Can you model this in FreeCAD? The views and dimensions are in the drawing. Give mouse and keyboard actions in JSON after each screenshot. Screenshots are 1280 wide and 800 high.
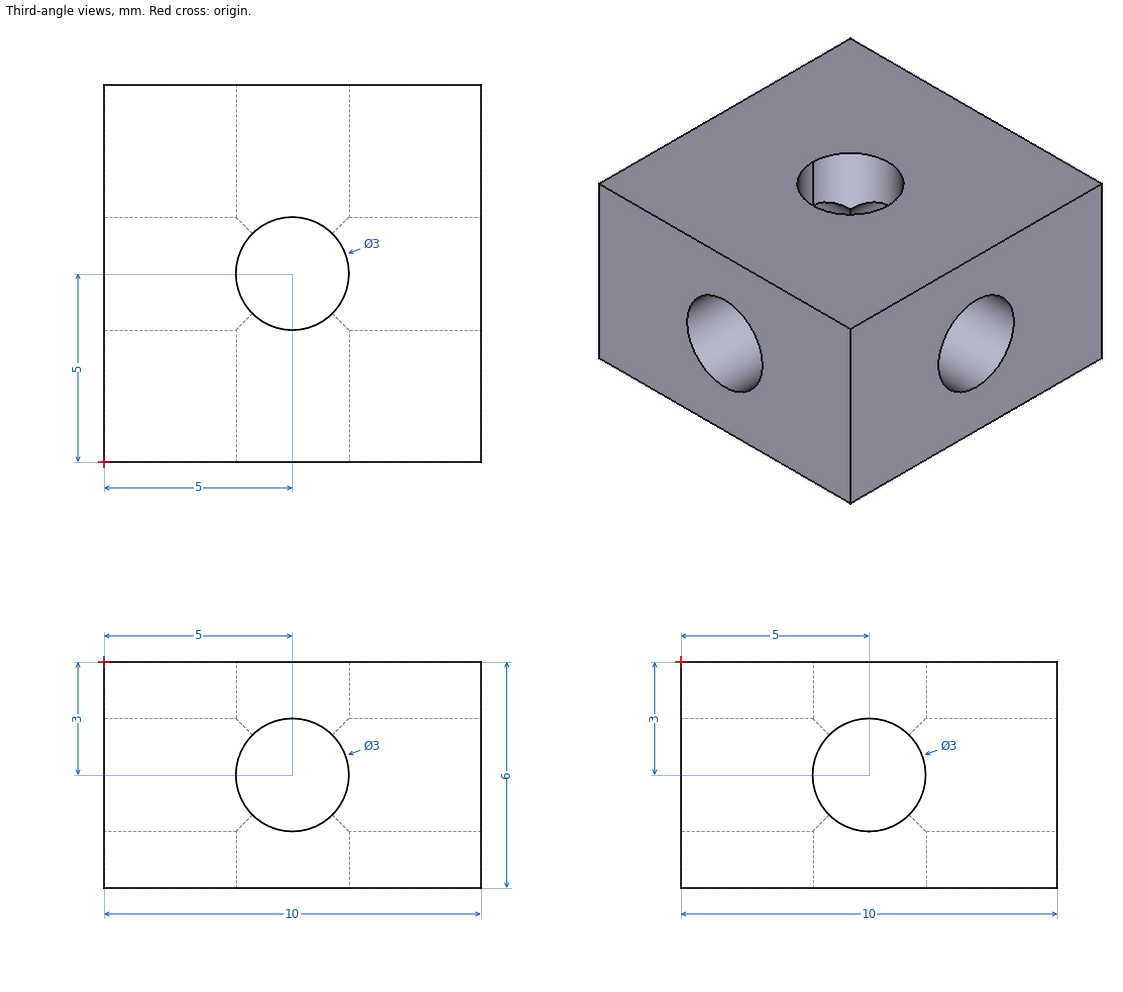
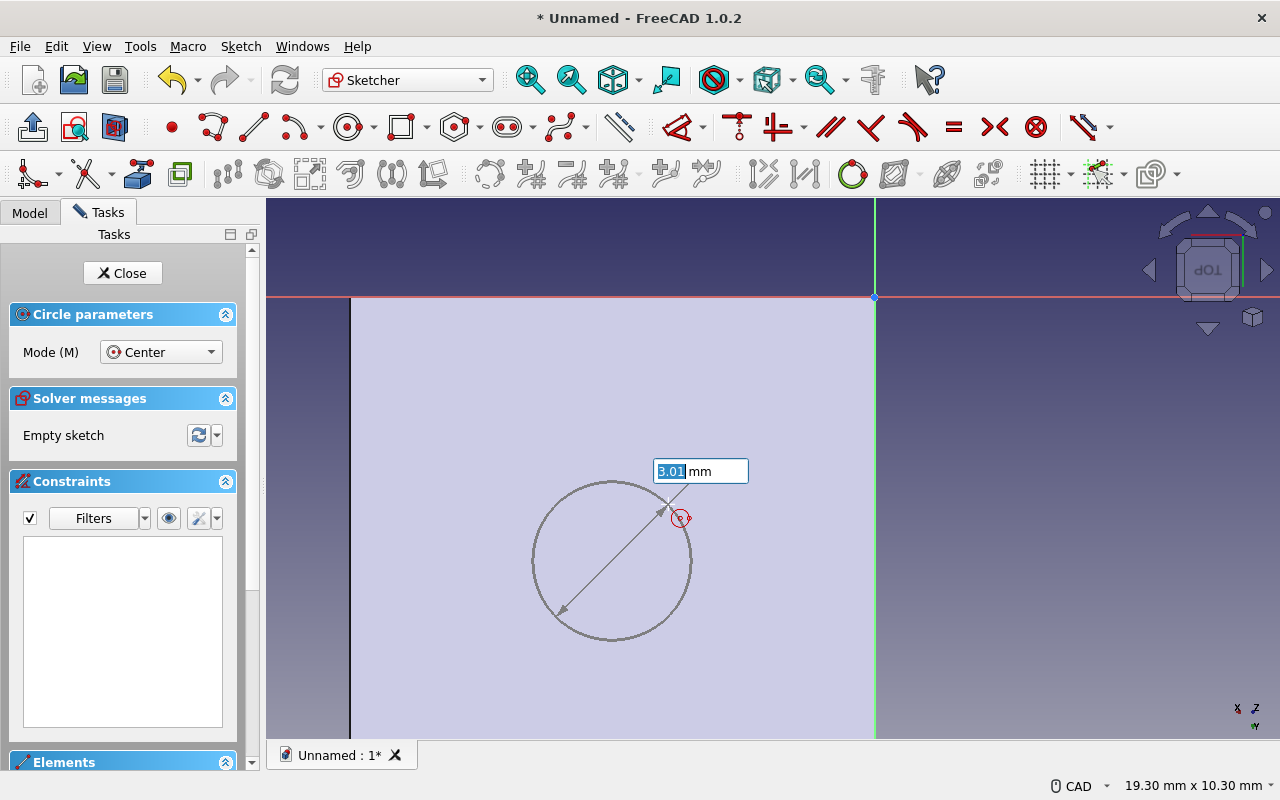
{"action": "type", "text": "3"}
{"action": "key", "text": "Return"}
{"action": "key", "text": "Escape"}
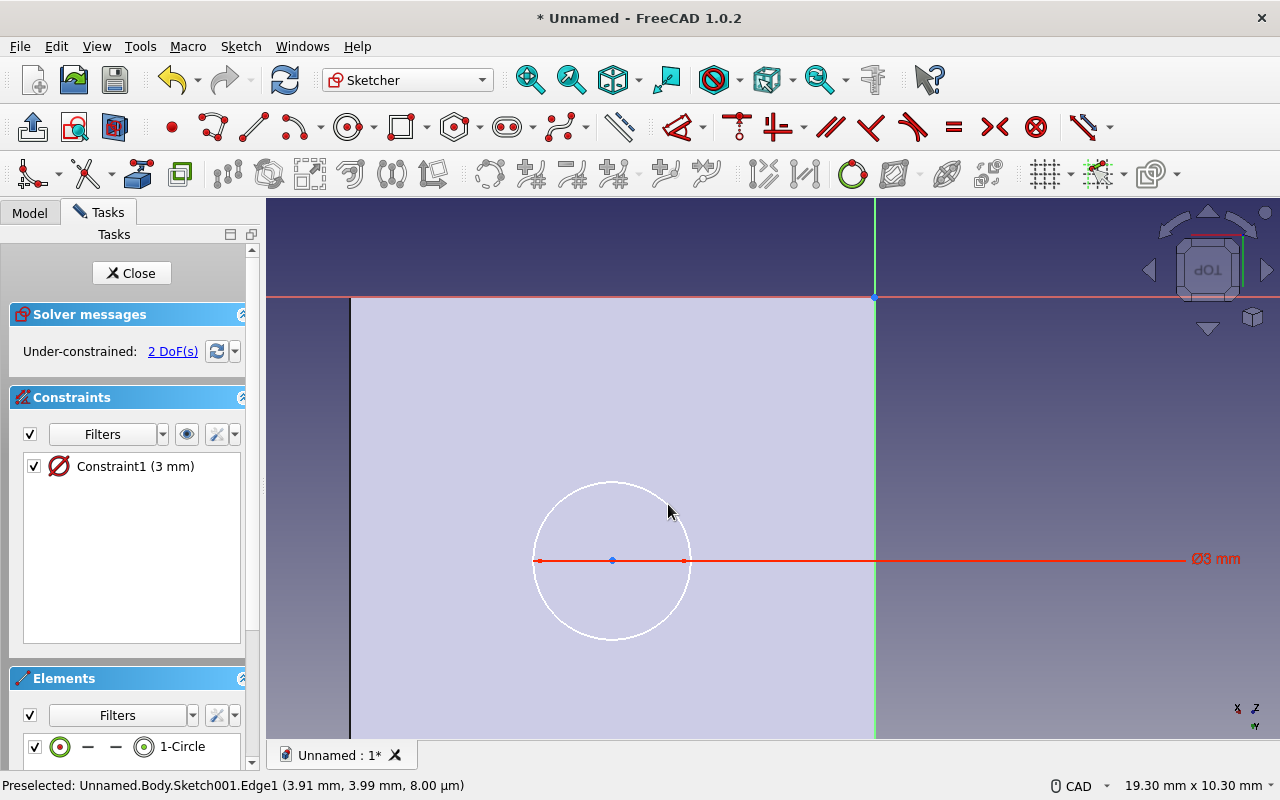
{"action": "left_click", "coordinate": [612, 561]}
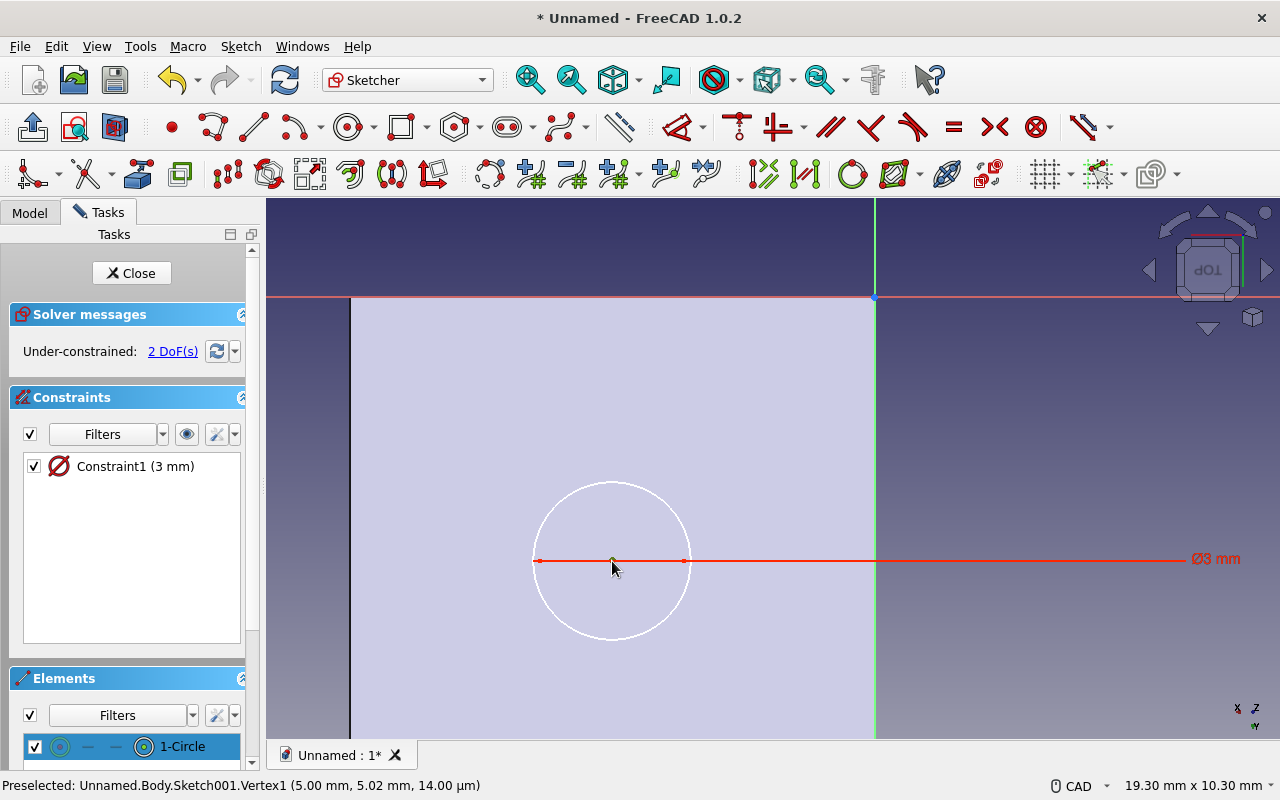
{"action": "key", "text": "l"}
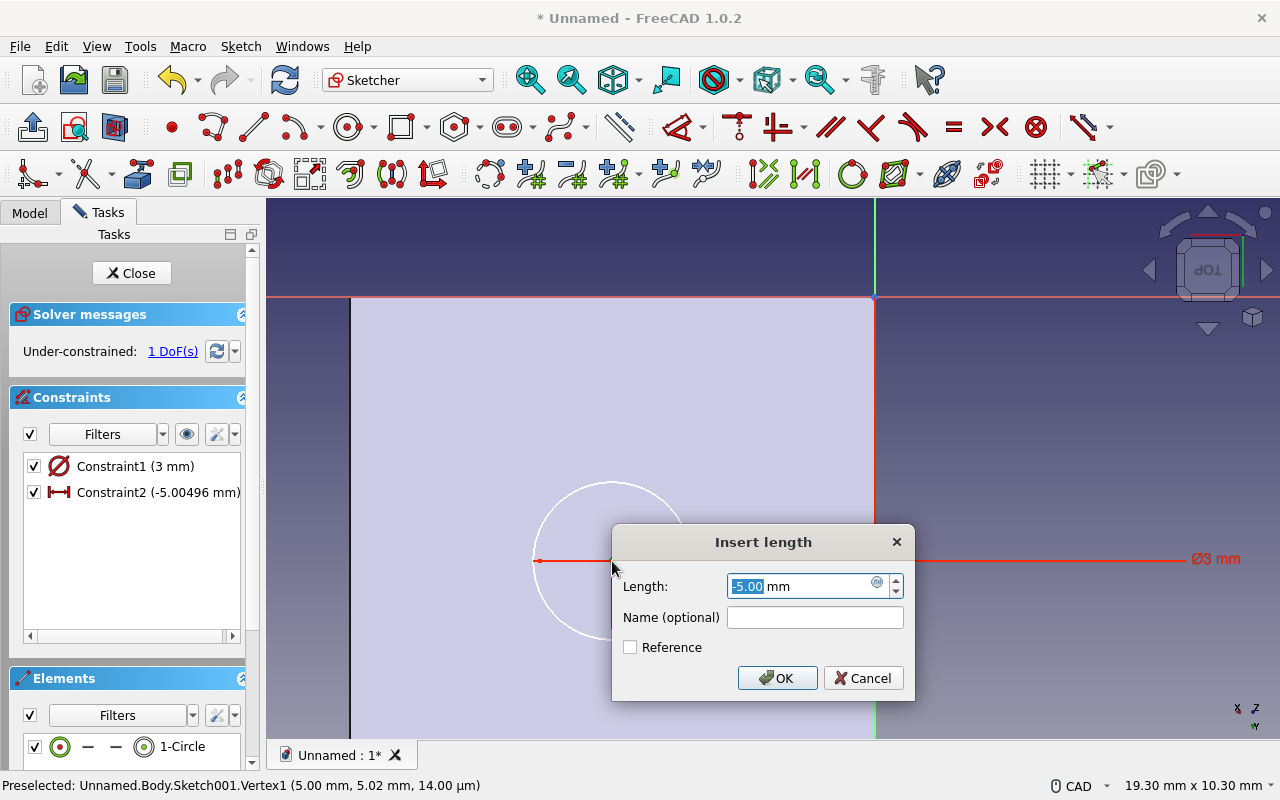
{"action": "type", "text": "-5"}
{"action": "key", "text": "Return"}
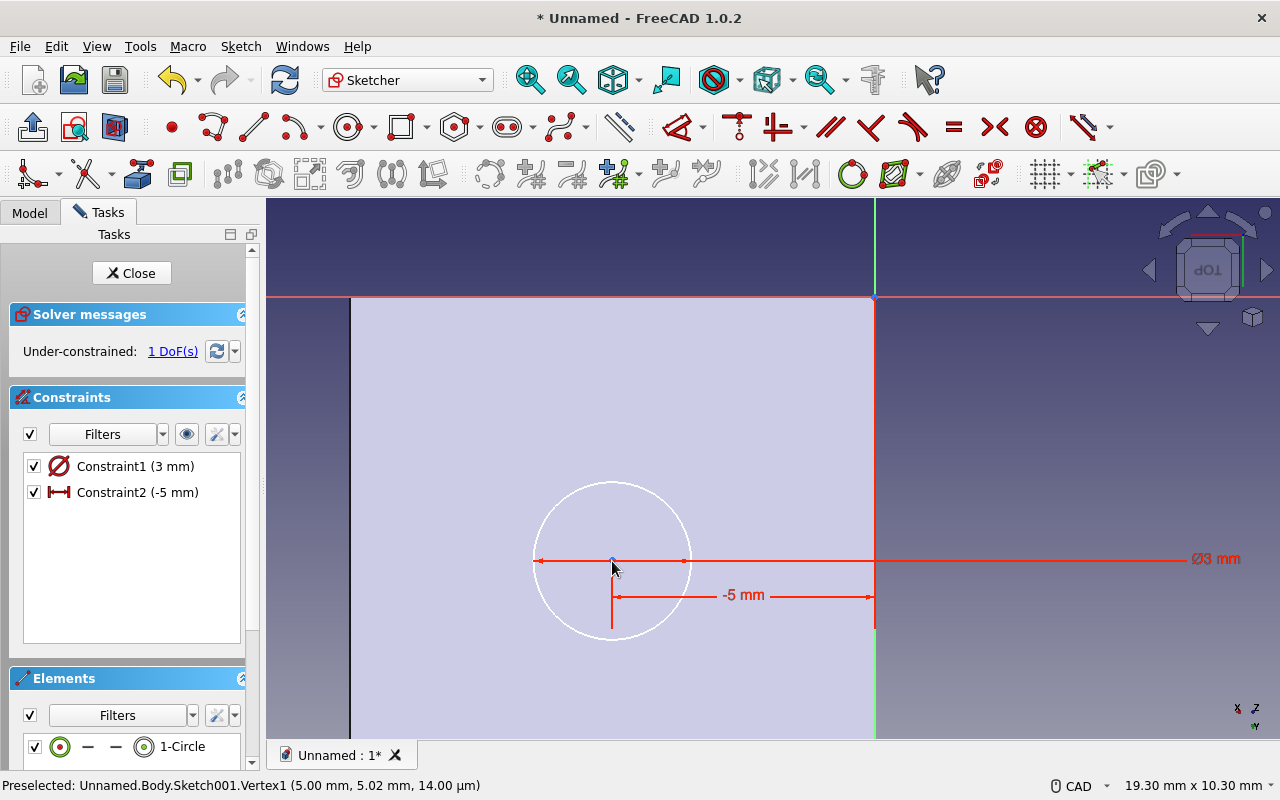
{"action": "left_click", "coordinate": [612, 561]}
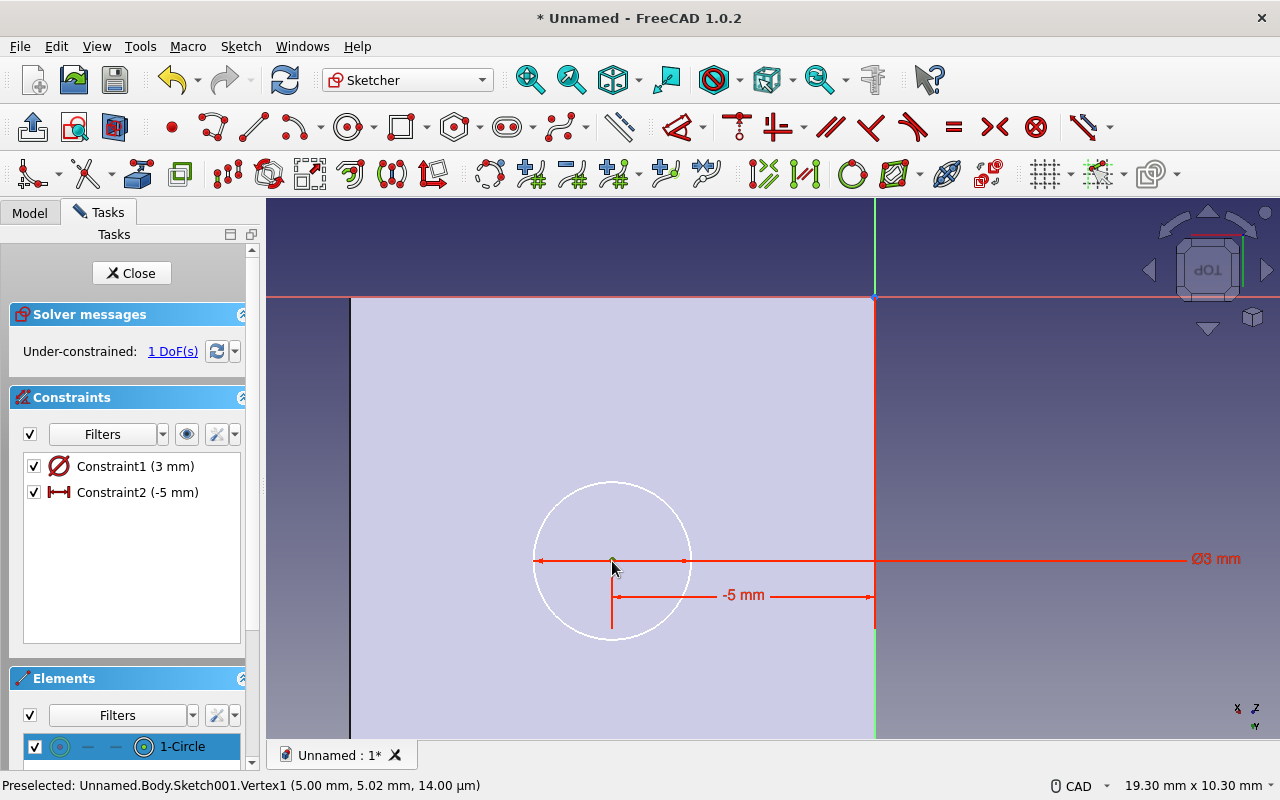
{"action": "left_click", "coordinate": [702, 128]}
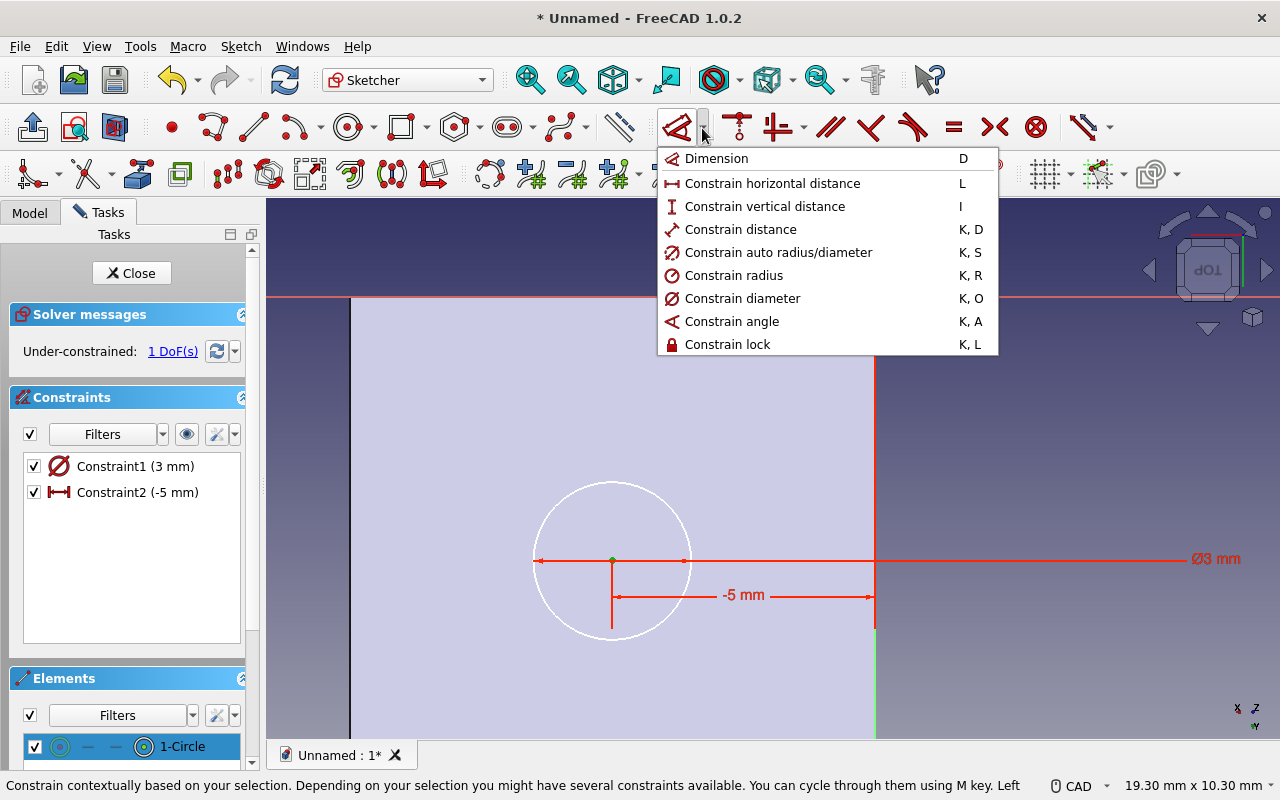
{"action": "left_click", "coordinate": [828, 206]}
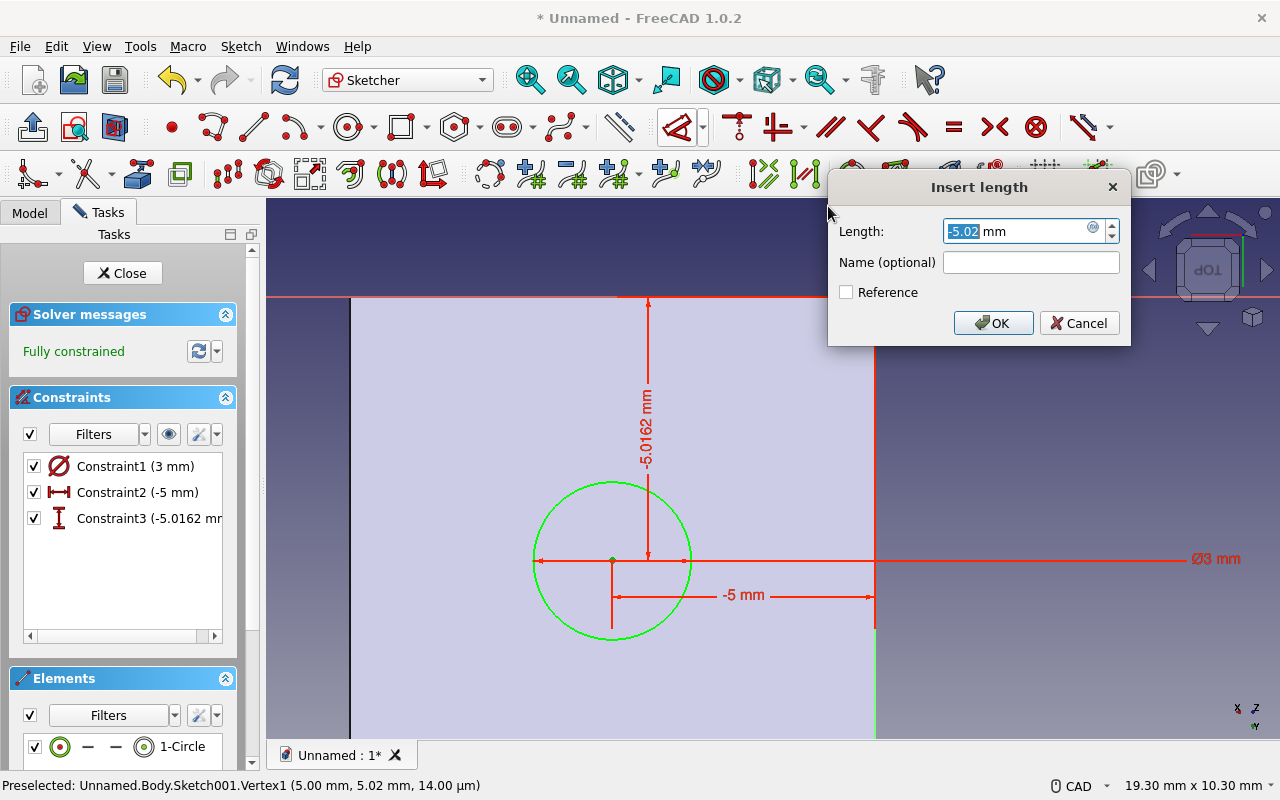
{"action": "type", "text": "-5"}
{"action": "key", "text": "Return"}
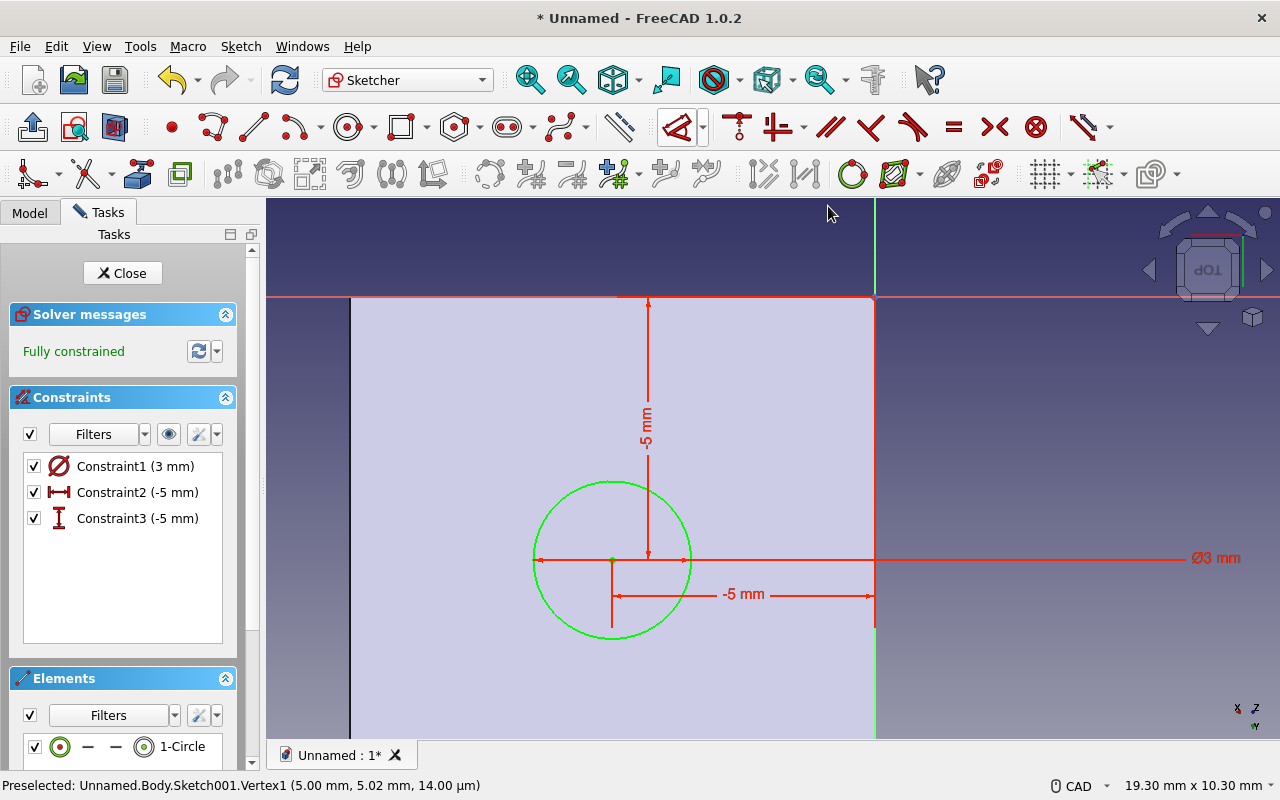
{"action": "left_click", "coordinate": [123, 273]}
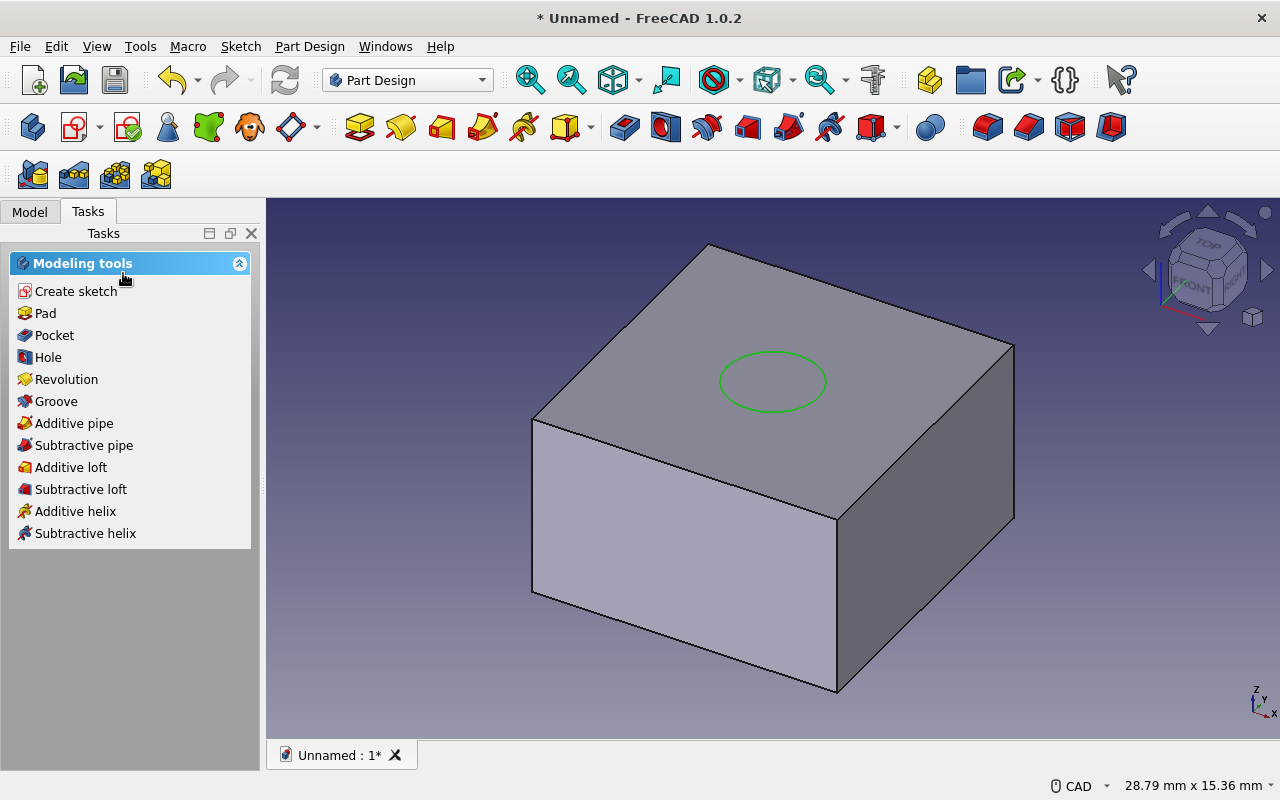
{"action": "left_click", "coordinate": [625, 128]}